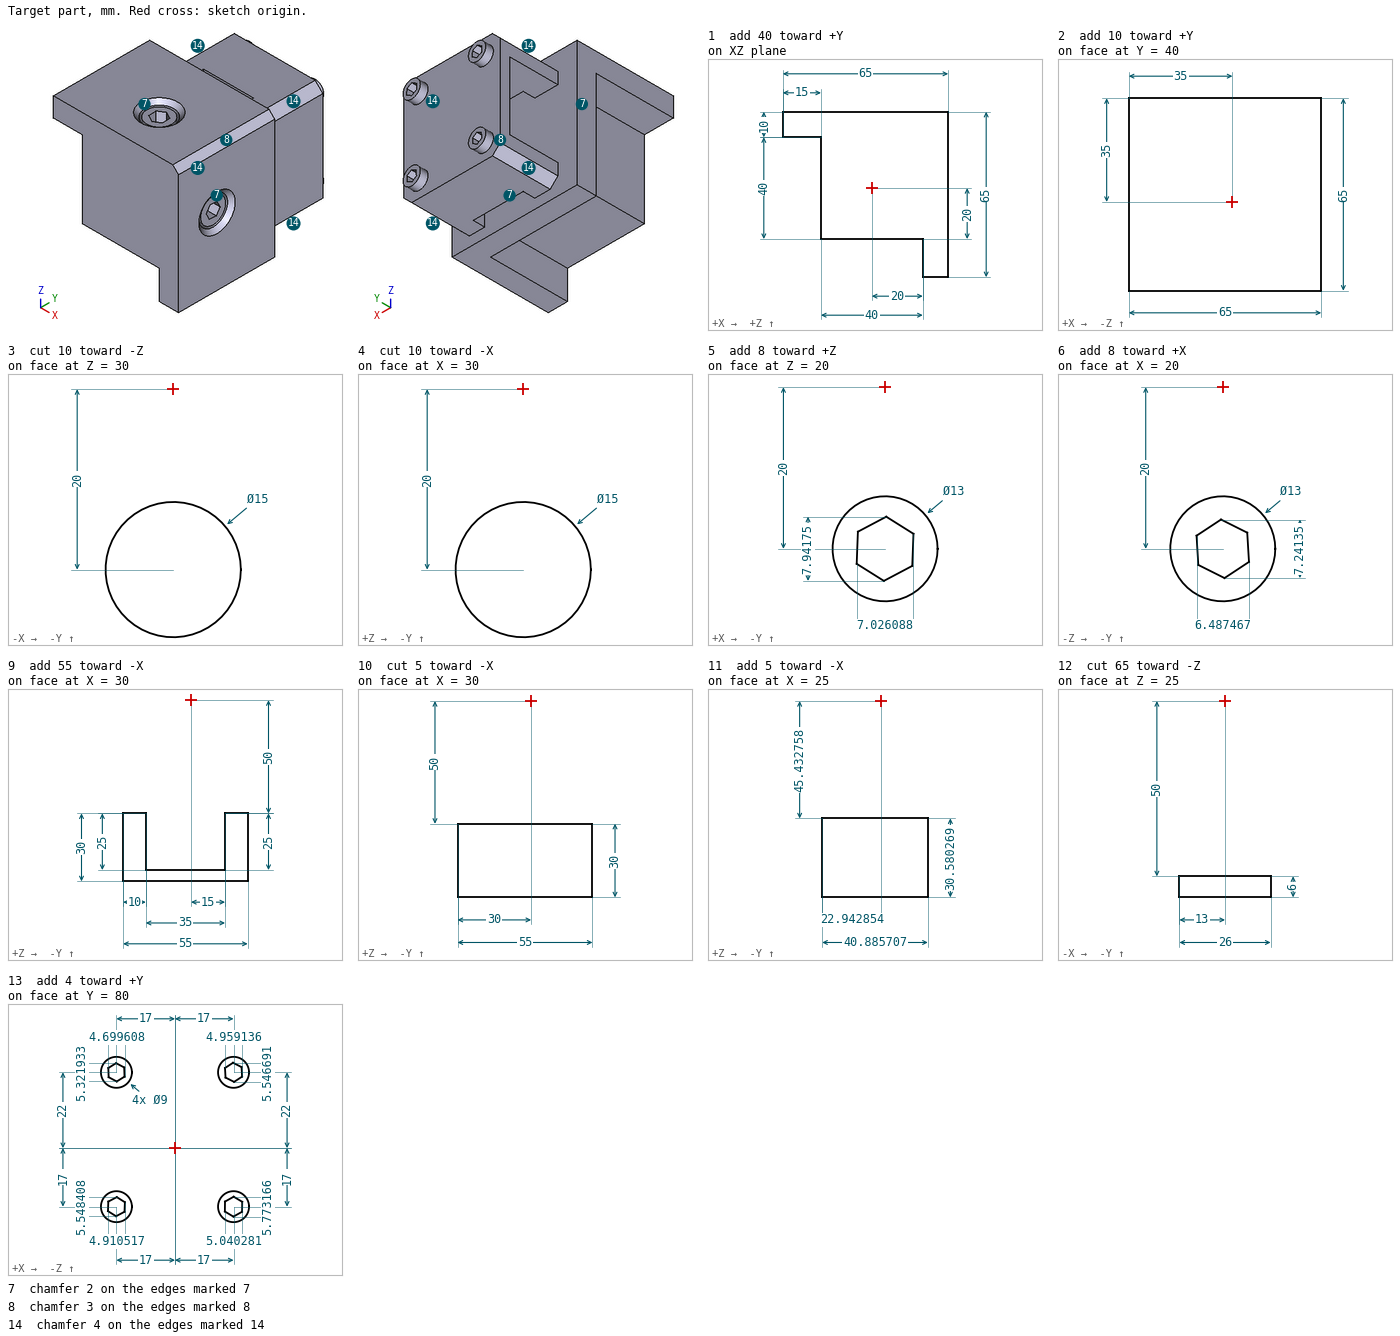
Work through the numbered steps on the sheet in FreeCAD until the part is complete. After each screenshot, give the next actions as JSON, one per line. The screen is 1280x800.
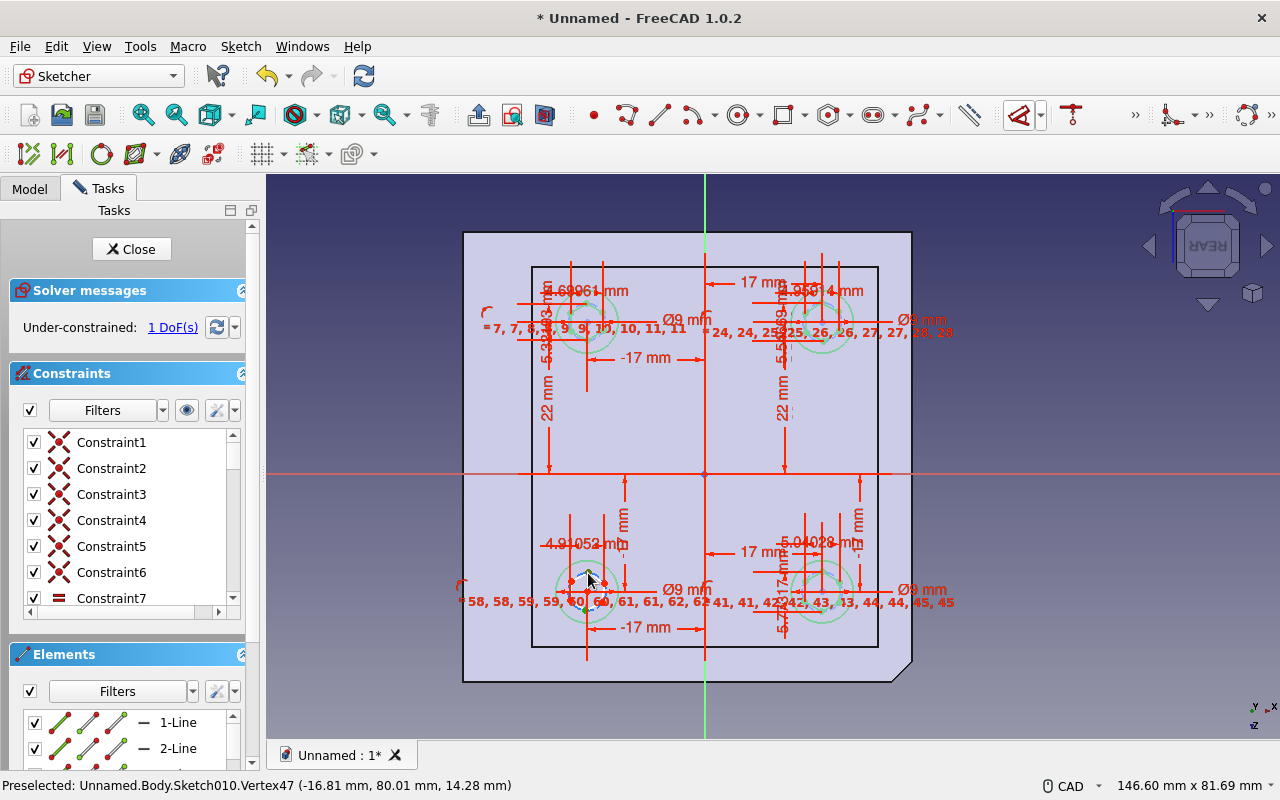
{"action": "key", "text": "i"}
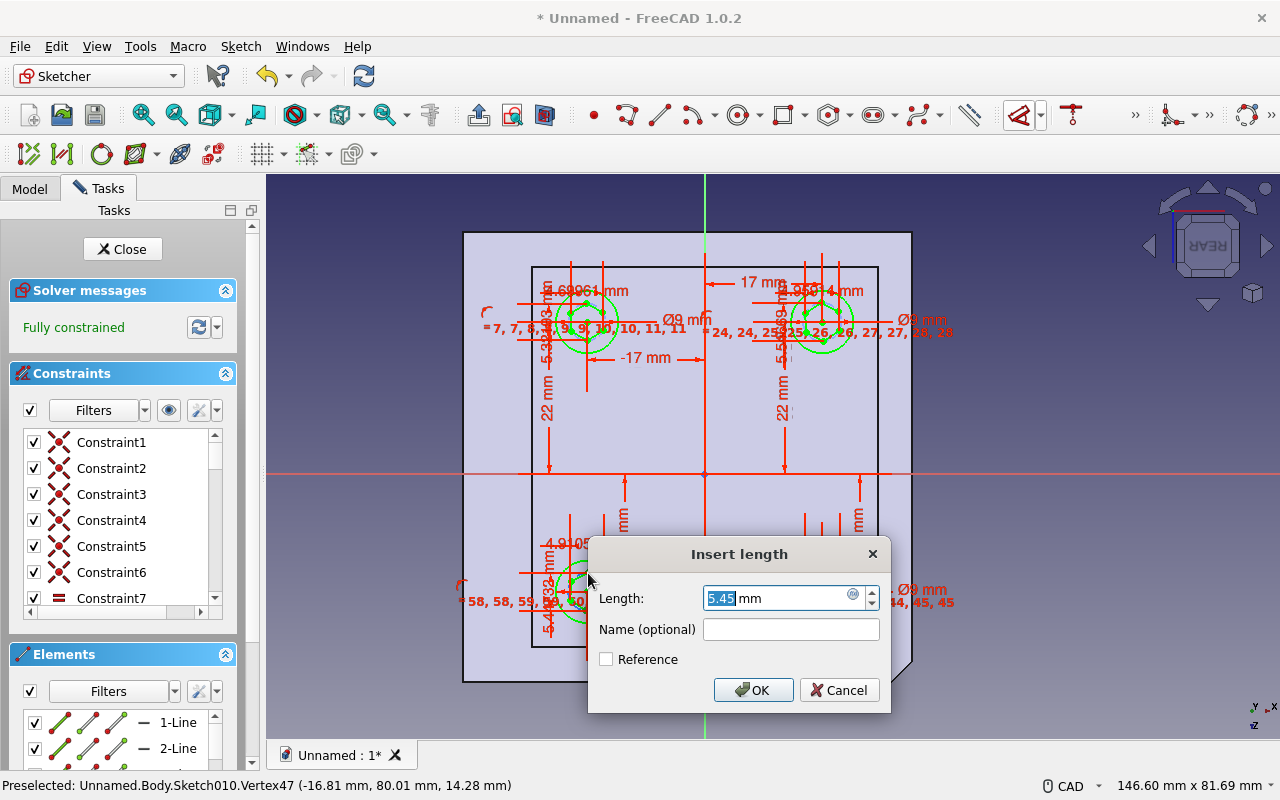
{"action": "type", "text": "5.548408"}
{"action": "key", "text": "Return"}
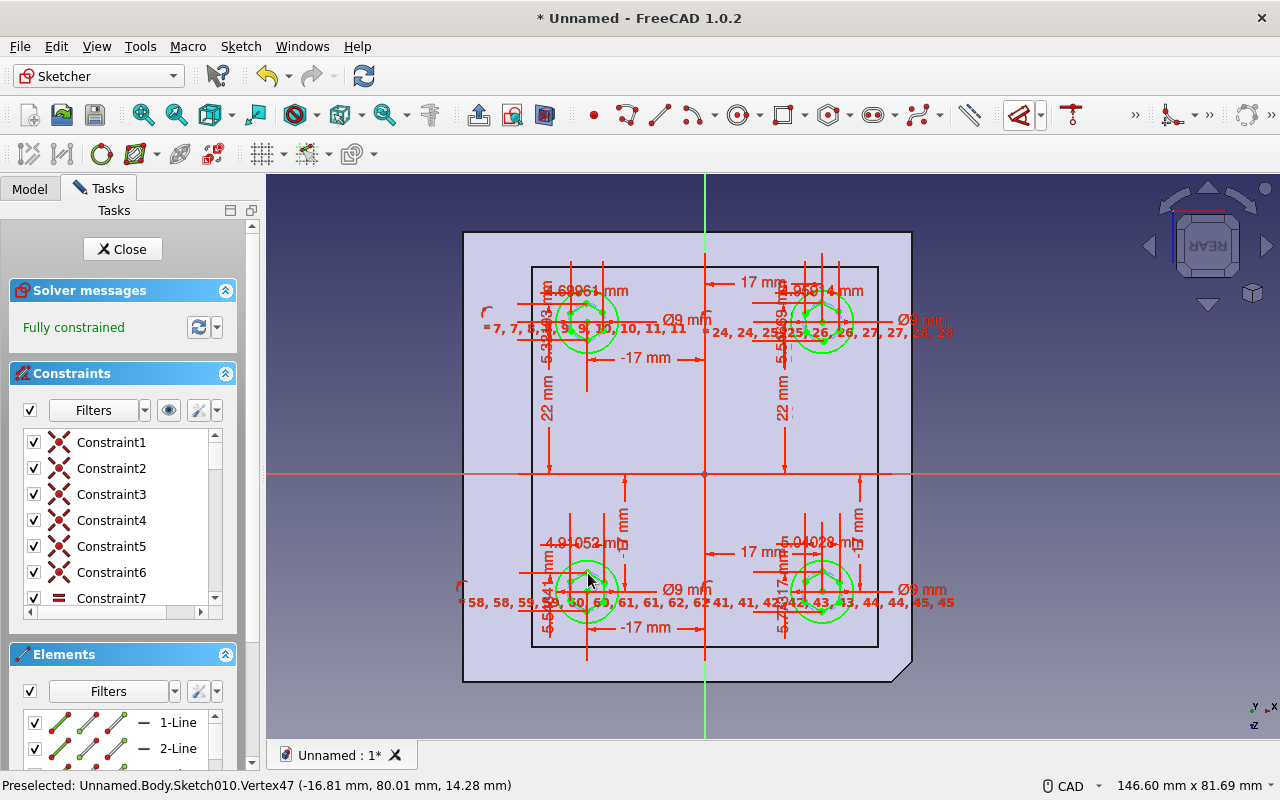
{"action": "left_click", "coordinate": [123, 249]}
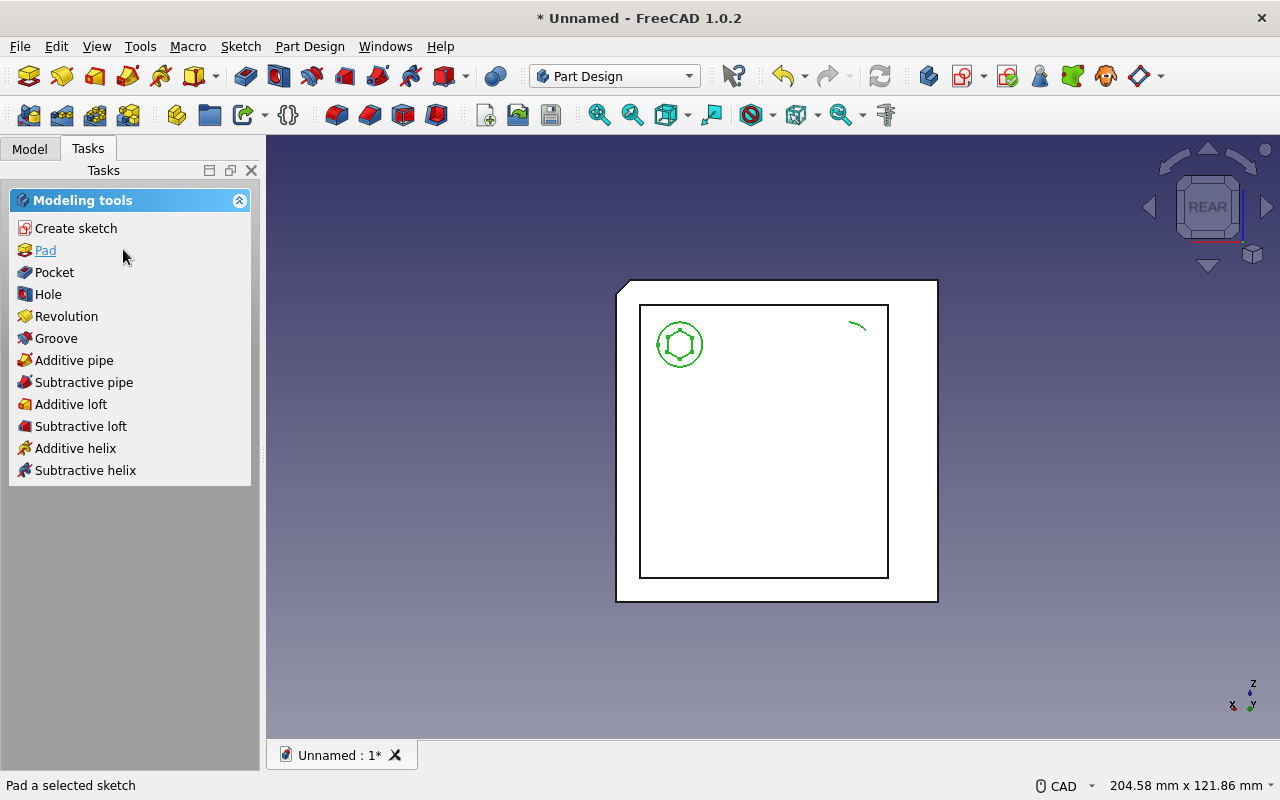
{"action": "left_click", "coordinate": [29, 76]}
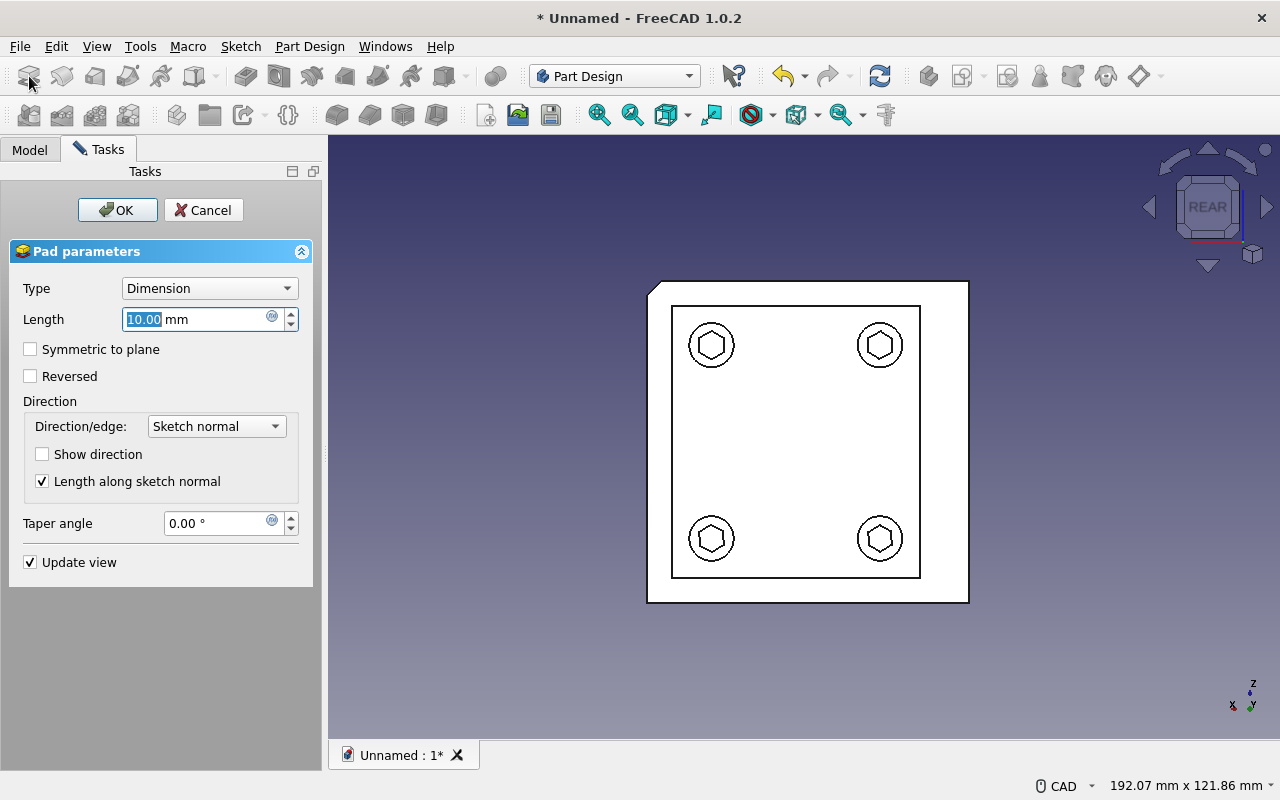
{"action": "type", "text": "4"}
{"action": "key", "text": "Tab"}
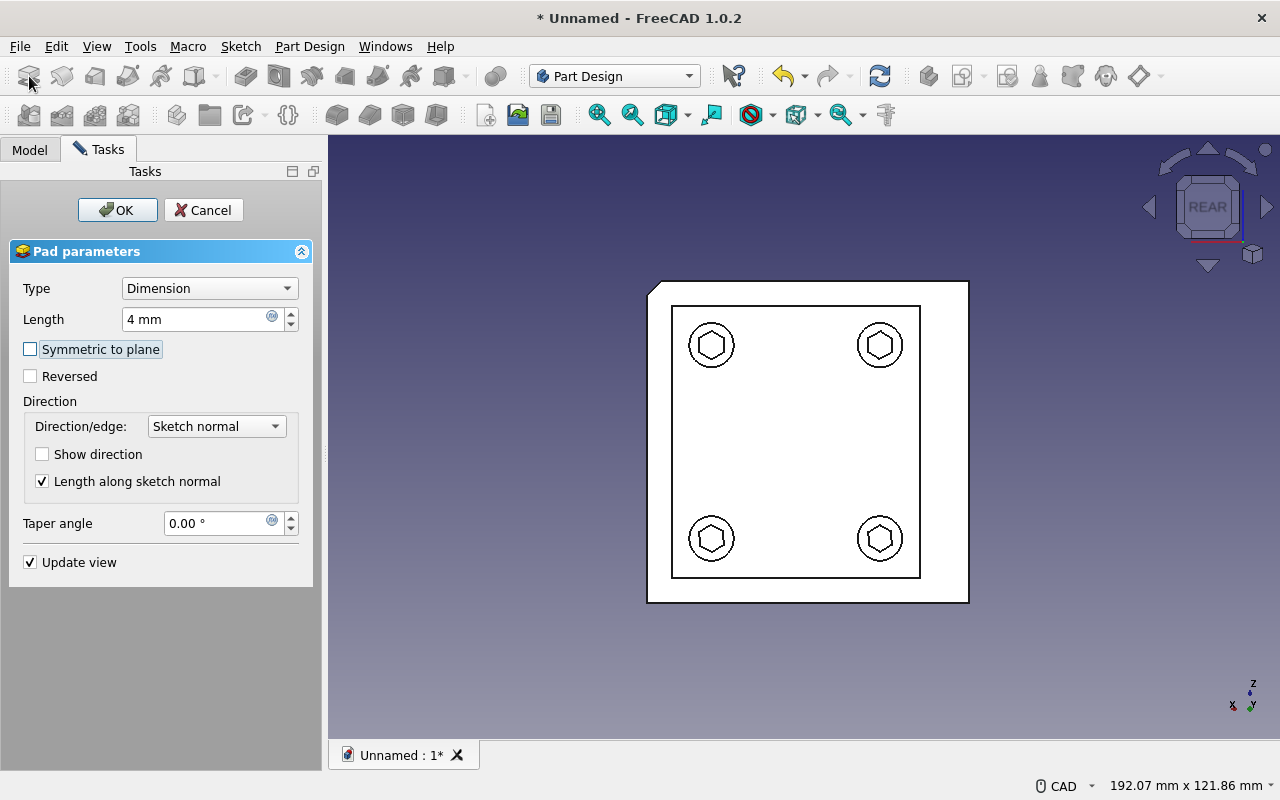
{"action": "left_click", "coordinate": [118, 210]}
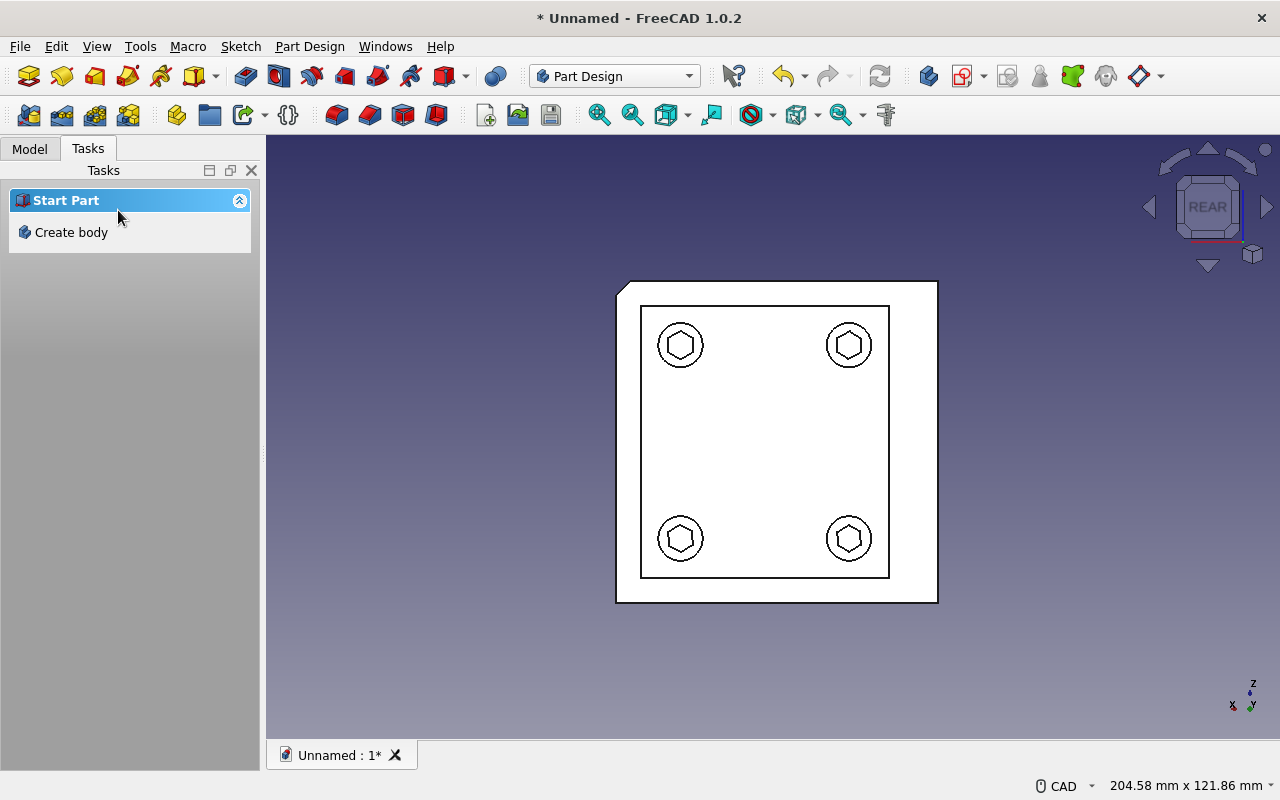
{"action": "key", "text": "0"}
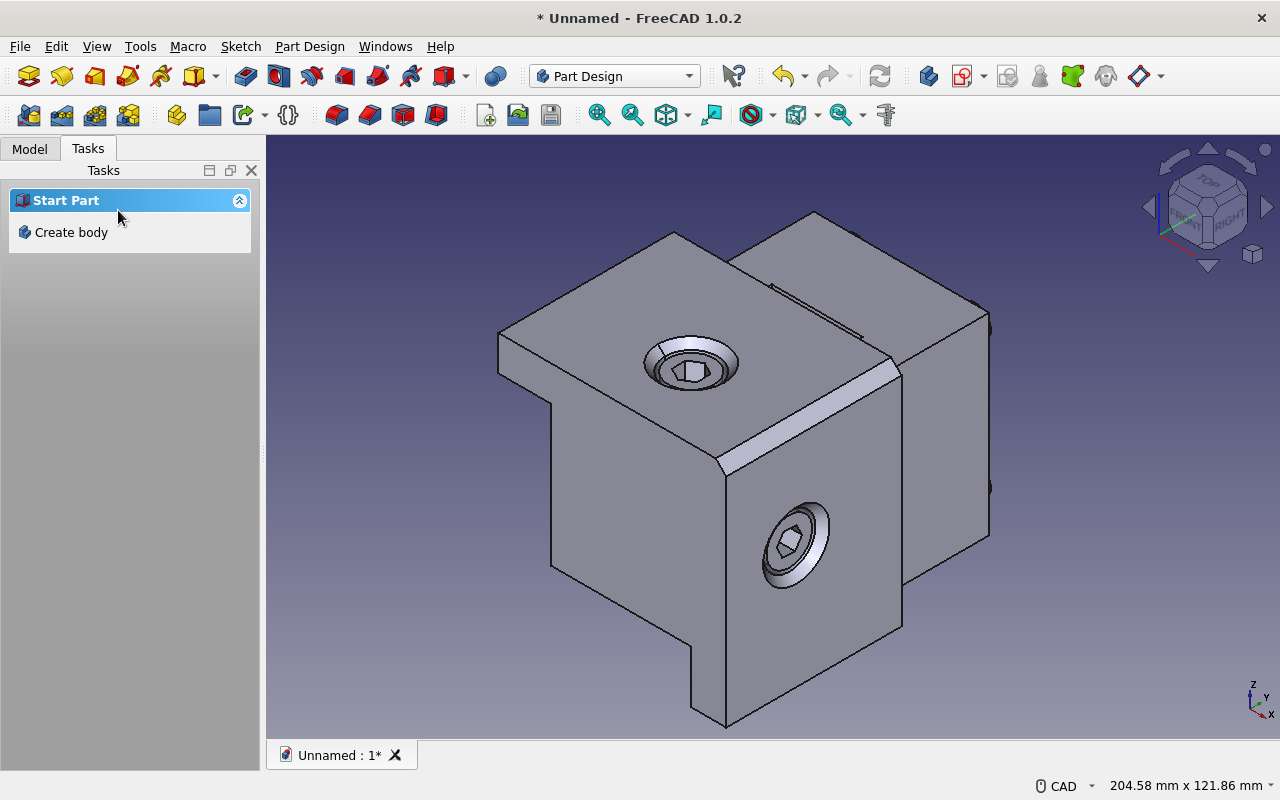
{"action": "left_click", "coordinate": [937, 342]}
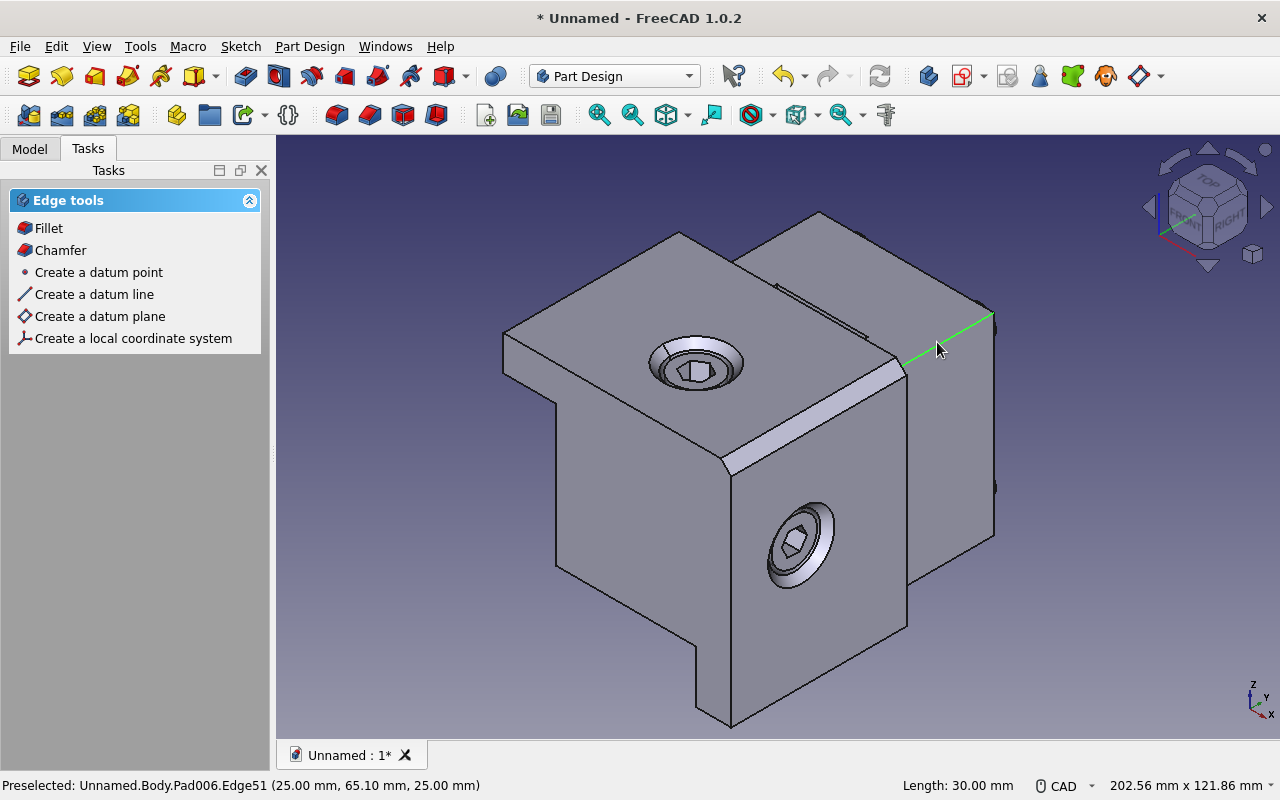
{"action": "key", "text": "2"}